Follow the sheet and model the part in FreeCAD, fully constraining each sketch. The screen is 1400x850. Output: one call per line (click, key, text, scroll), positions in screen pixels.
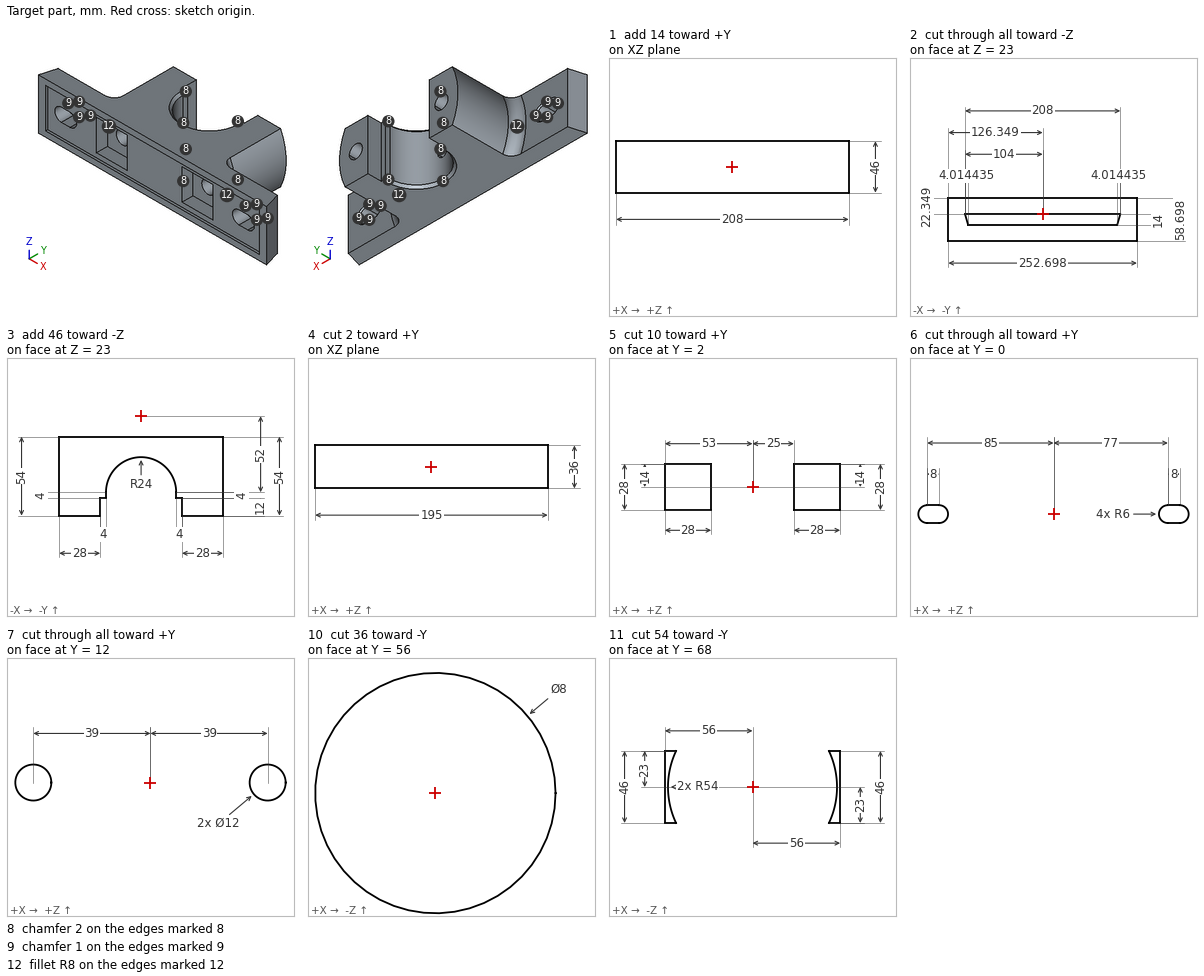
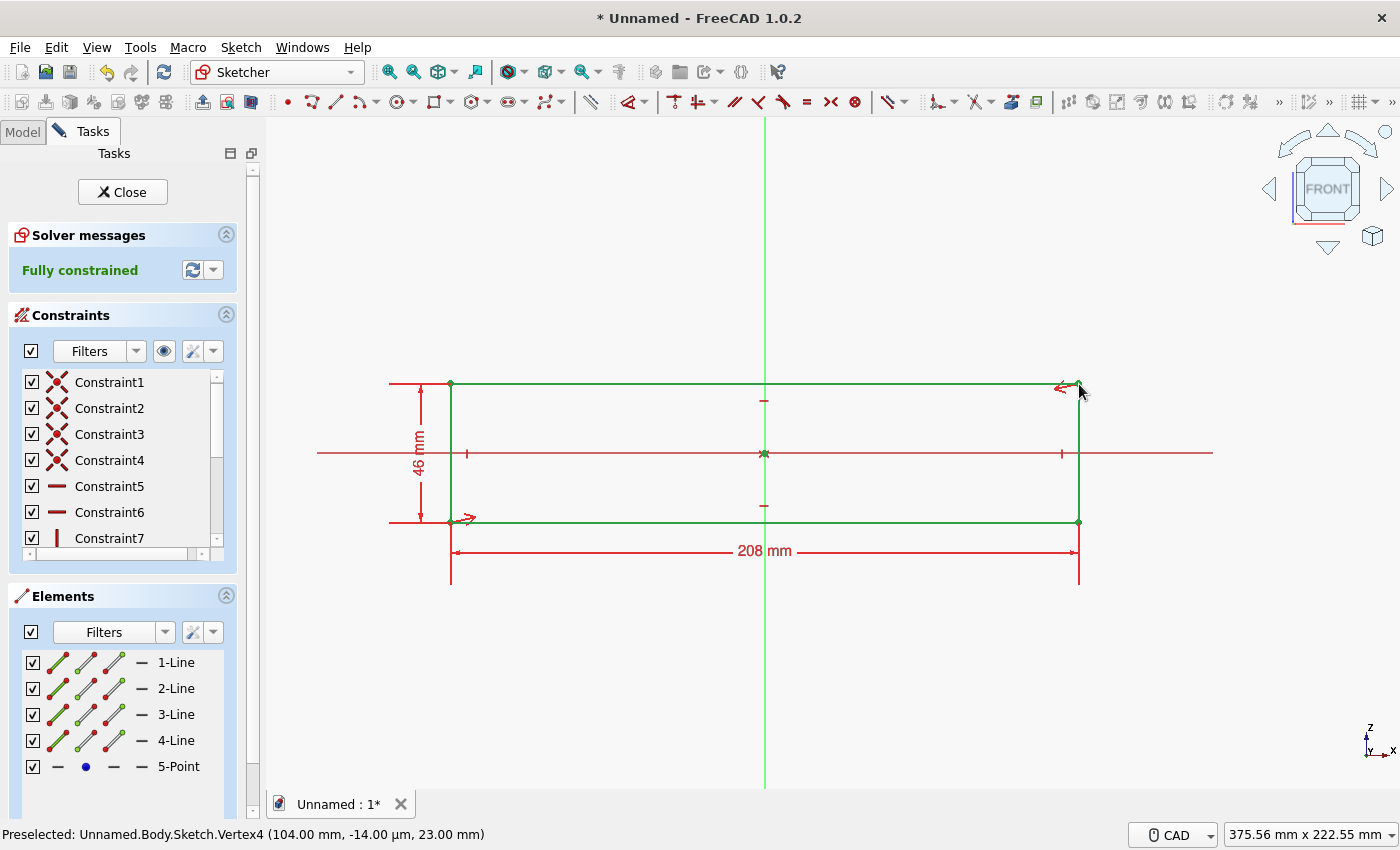
click(123, 192)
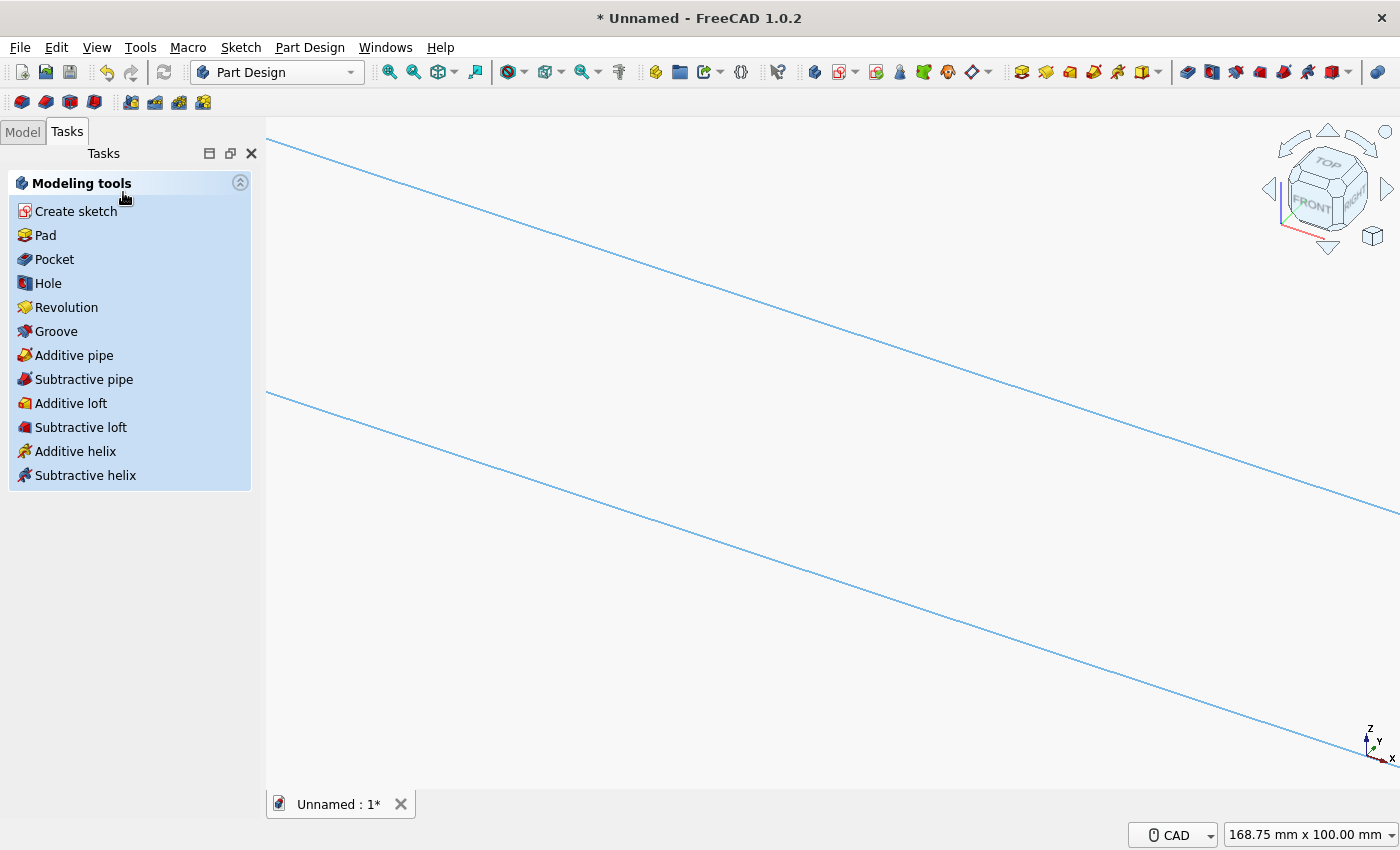
click(1022, 72)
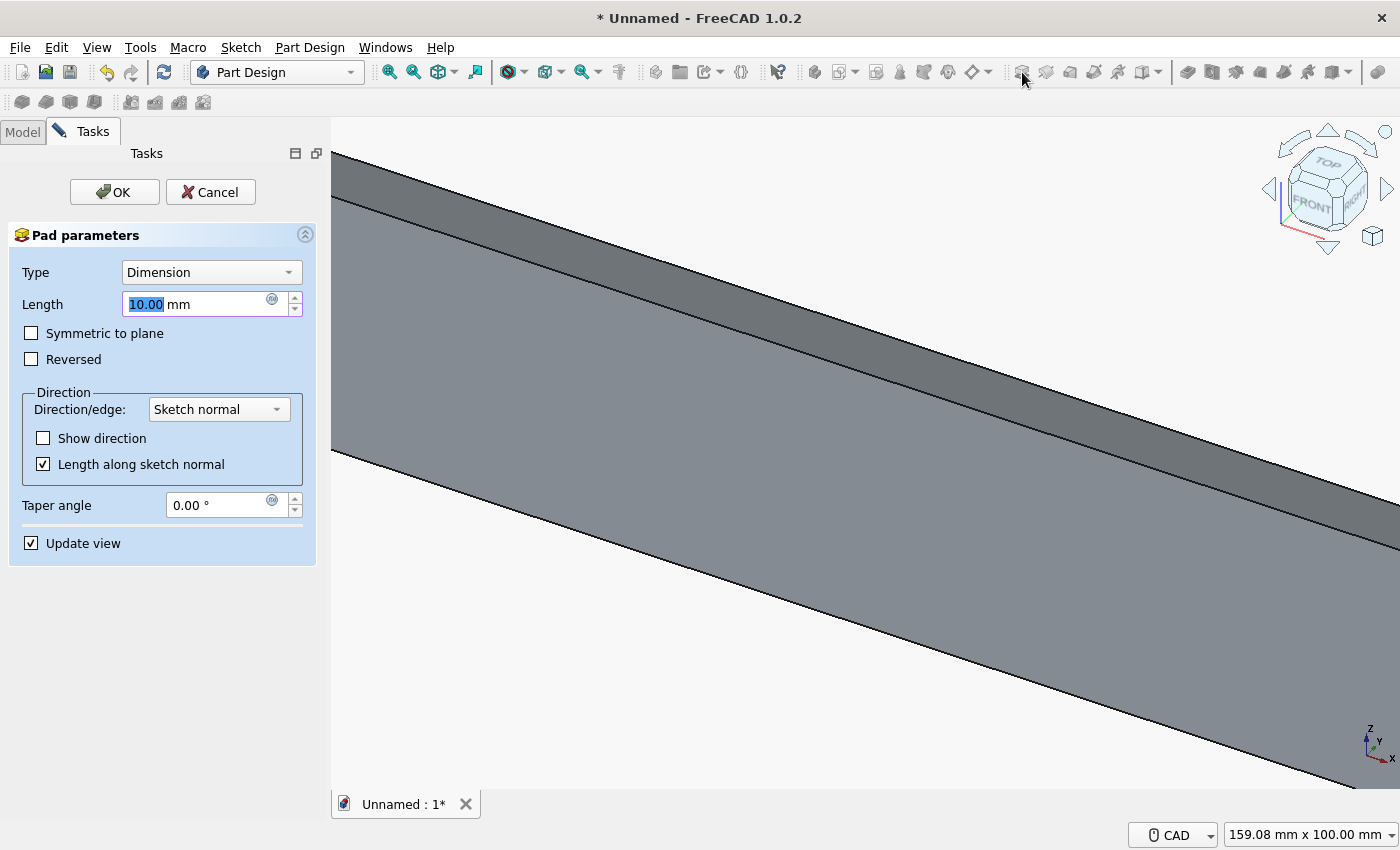
text(14)
key(Tab)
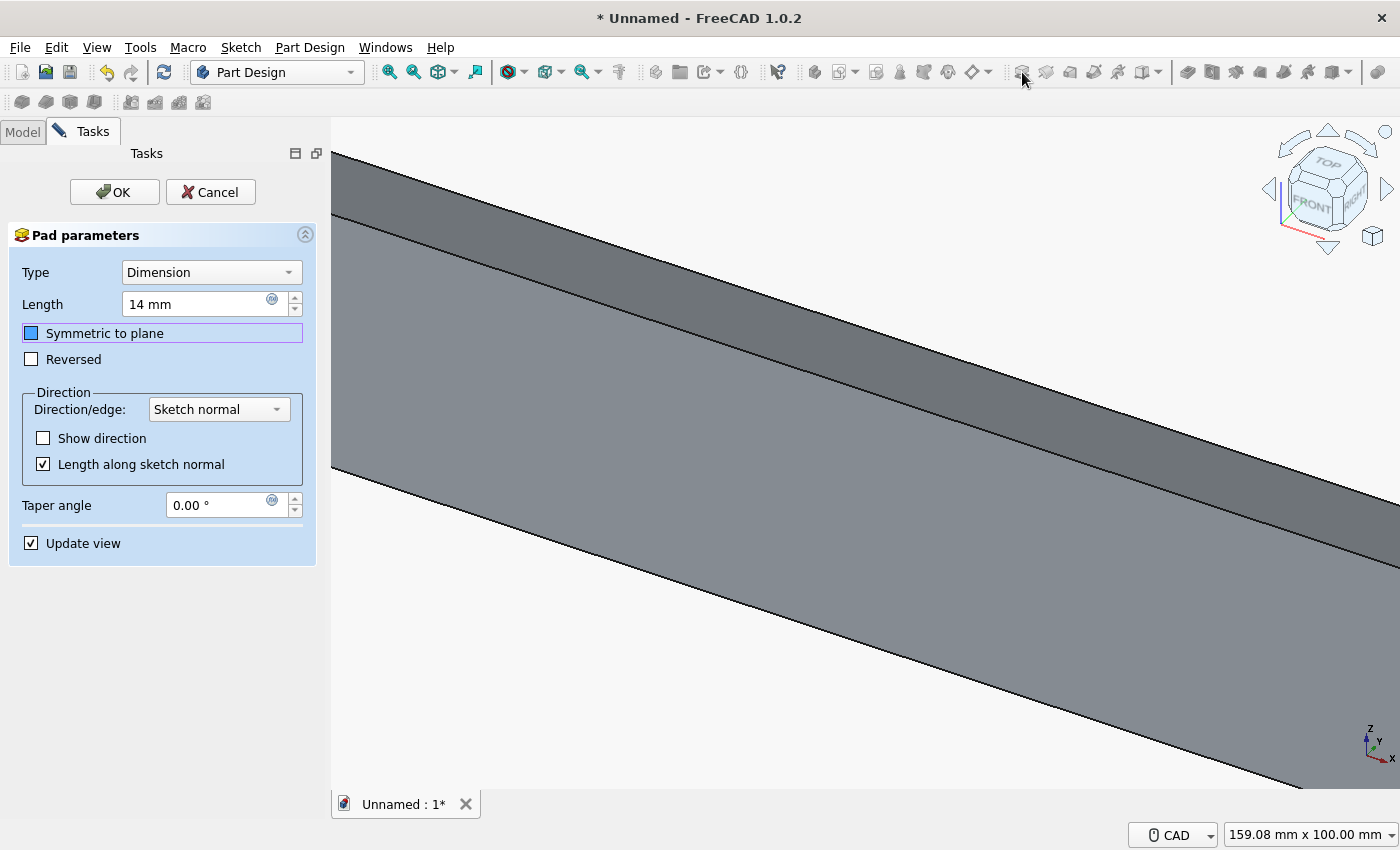
click(30, 359)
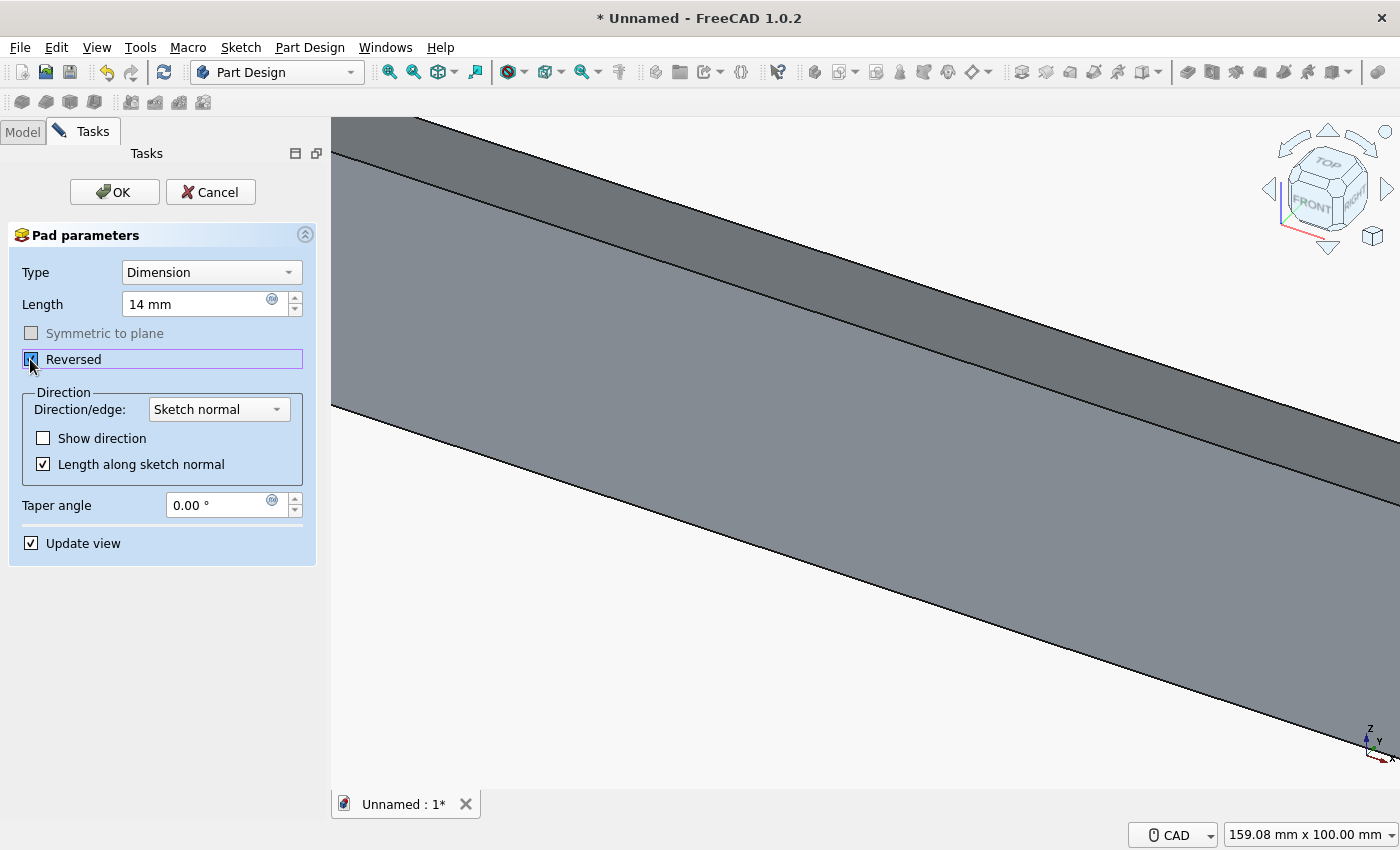
click(115, 192)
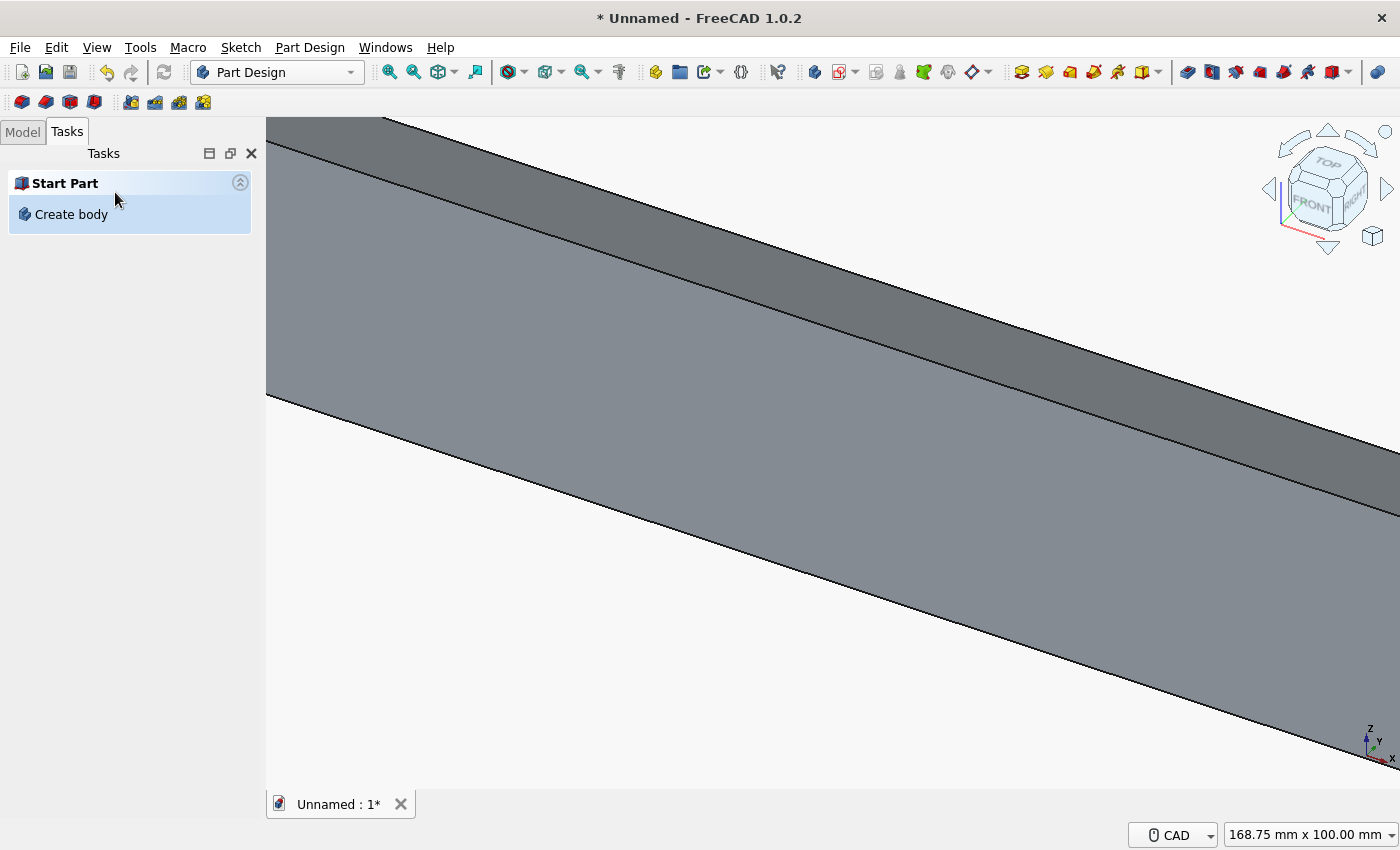
key(v)
key(f)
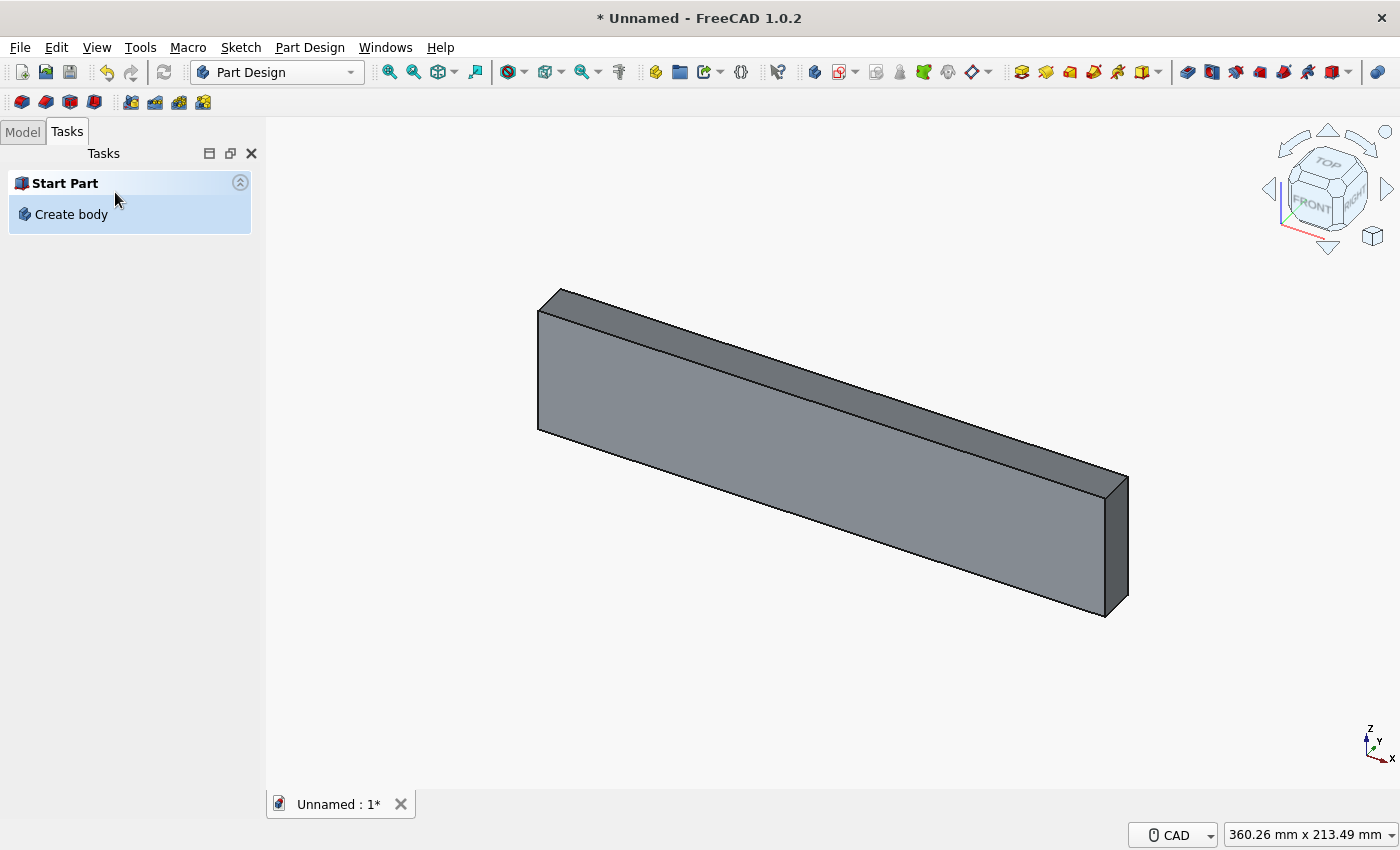
click(1076, 473)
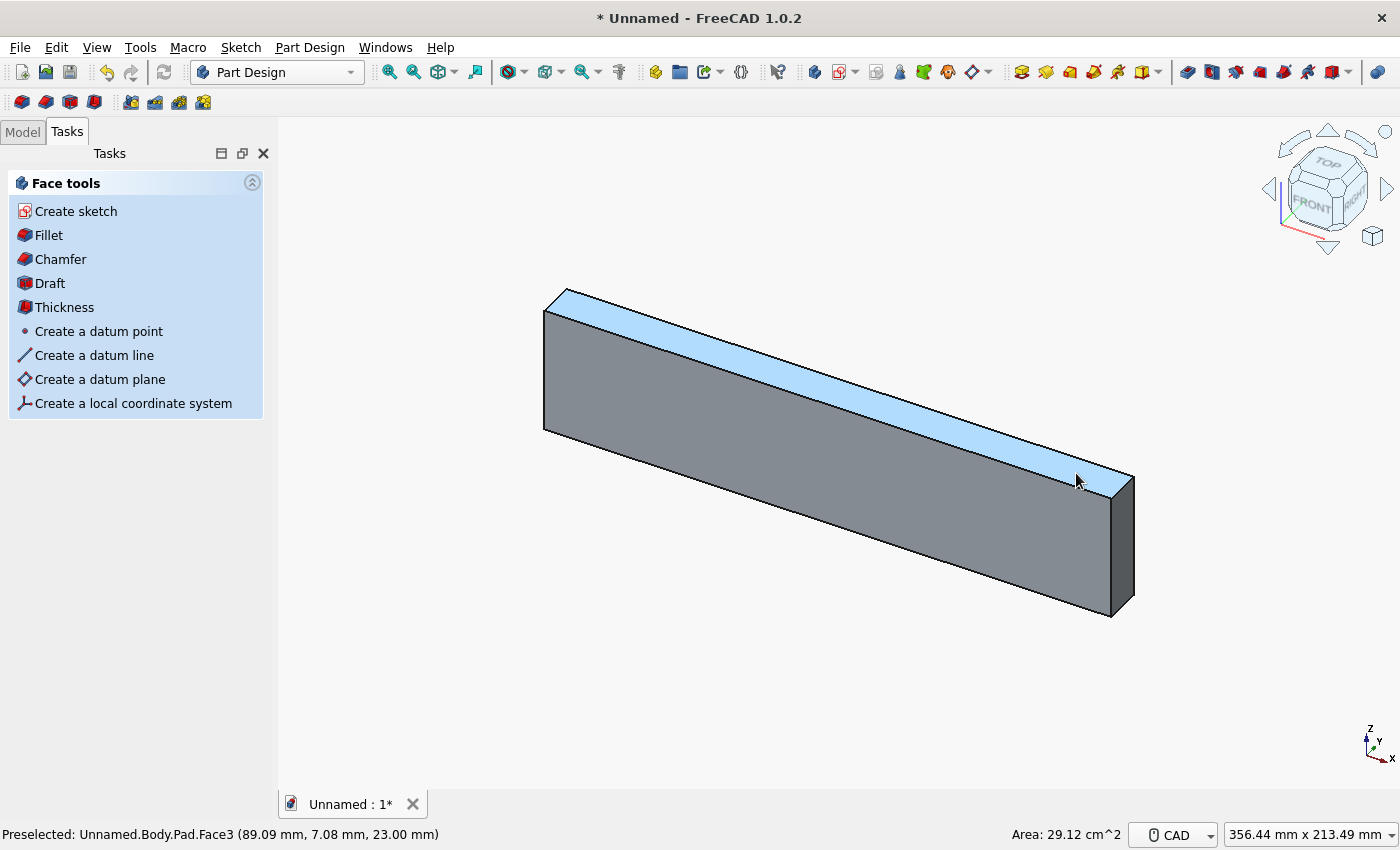
click(840, 72)